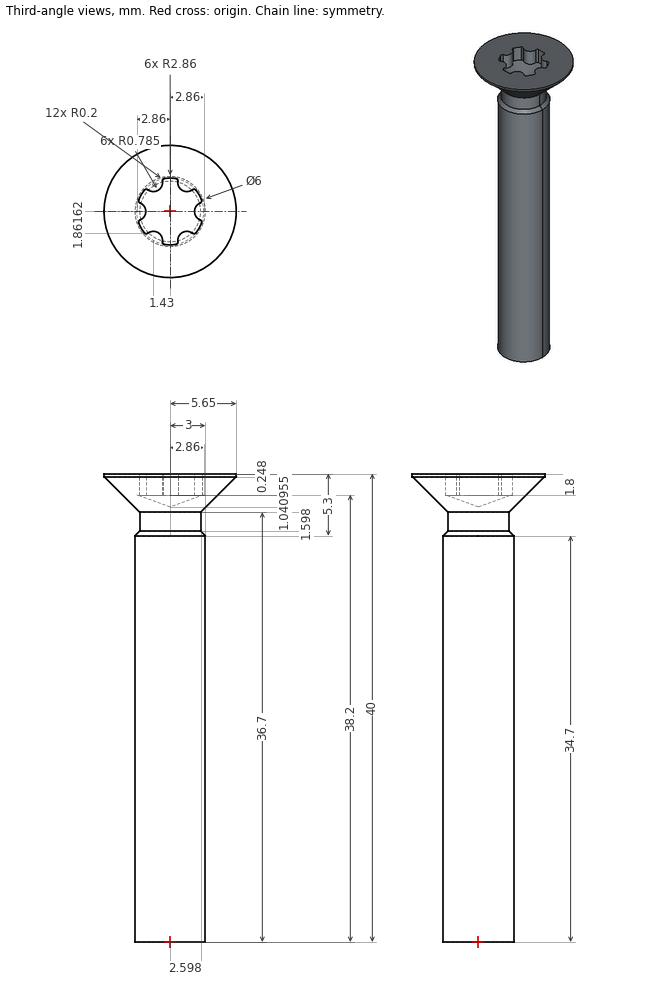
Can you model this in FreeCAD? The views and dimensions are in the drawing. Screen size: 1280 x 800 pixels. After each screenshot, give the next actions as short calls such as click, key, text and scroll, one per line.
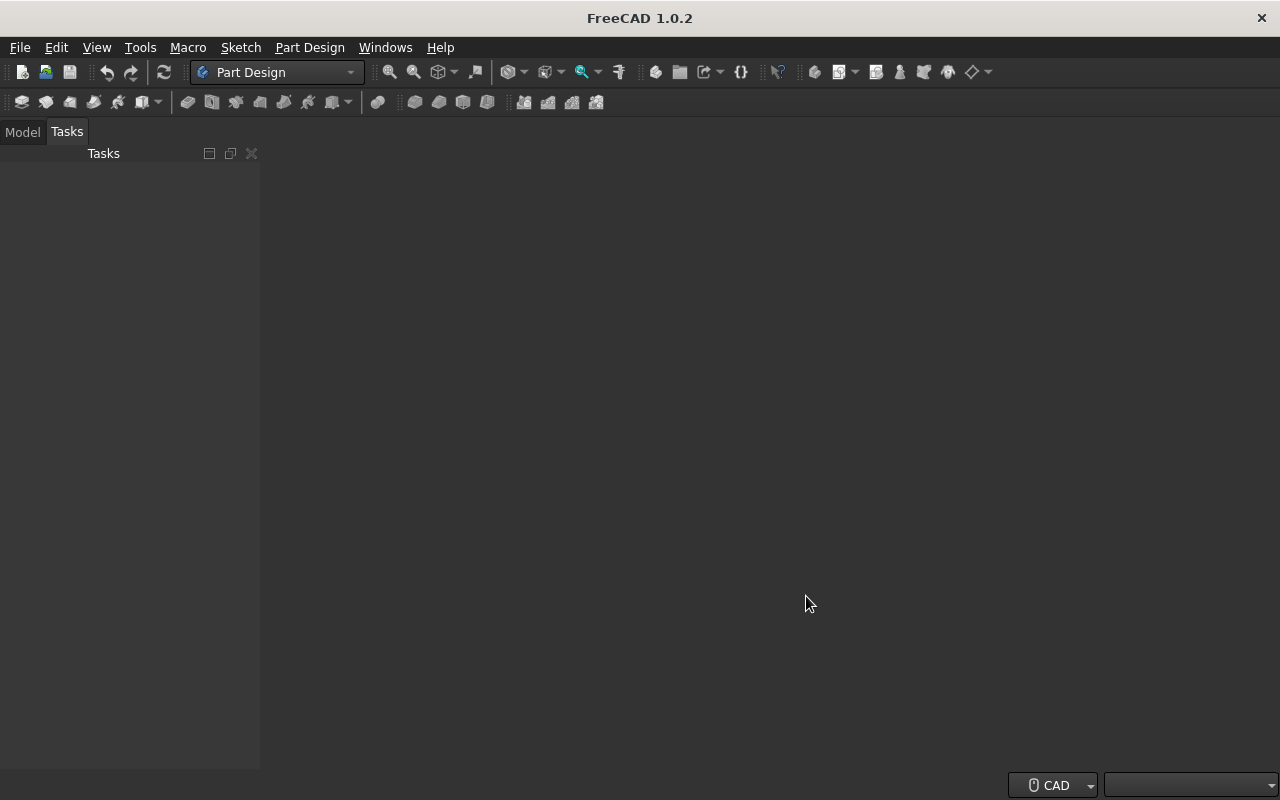
click(22, 72)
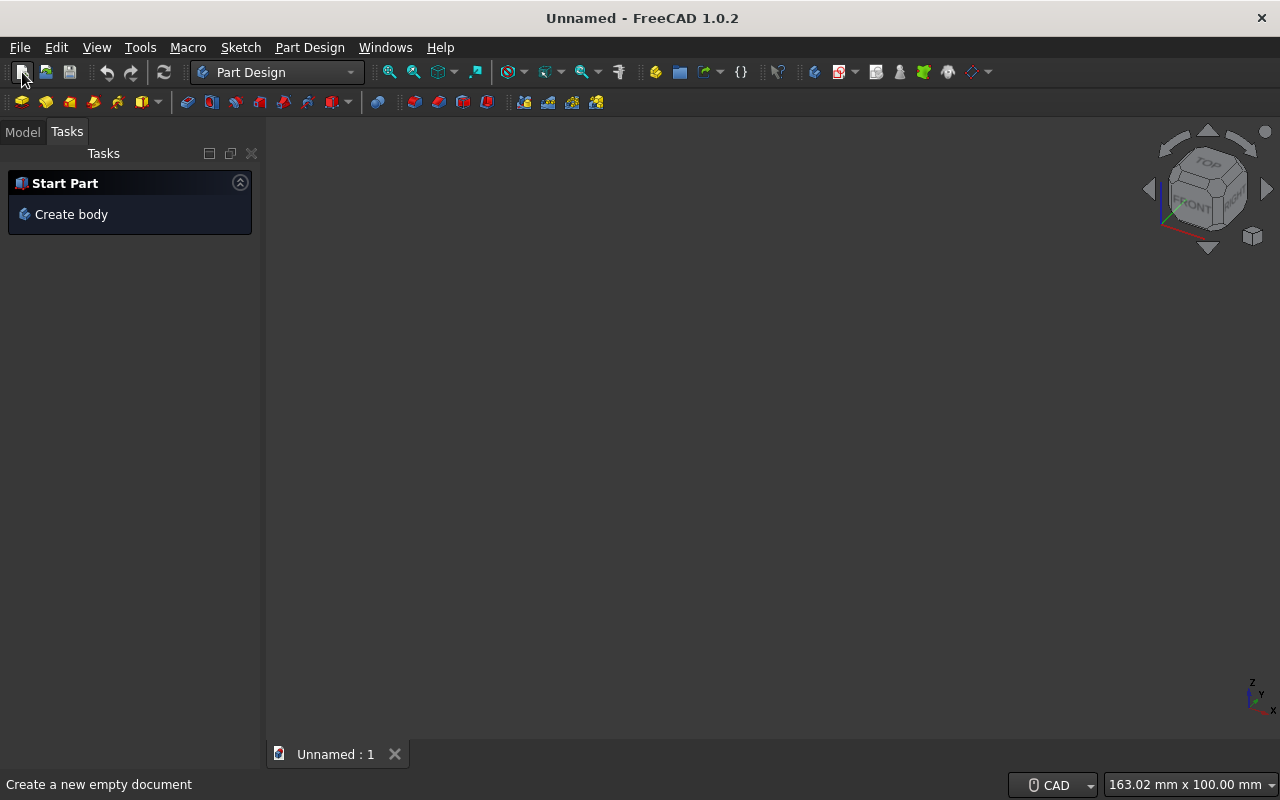
click(840, 72)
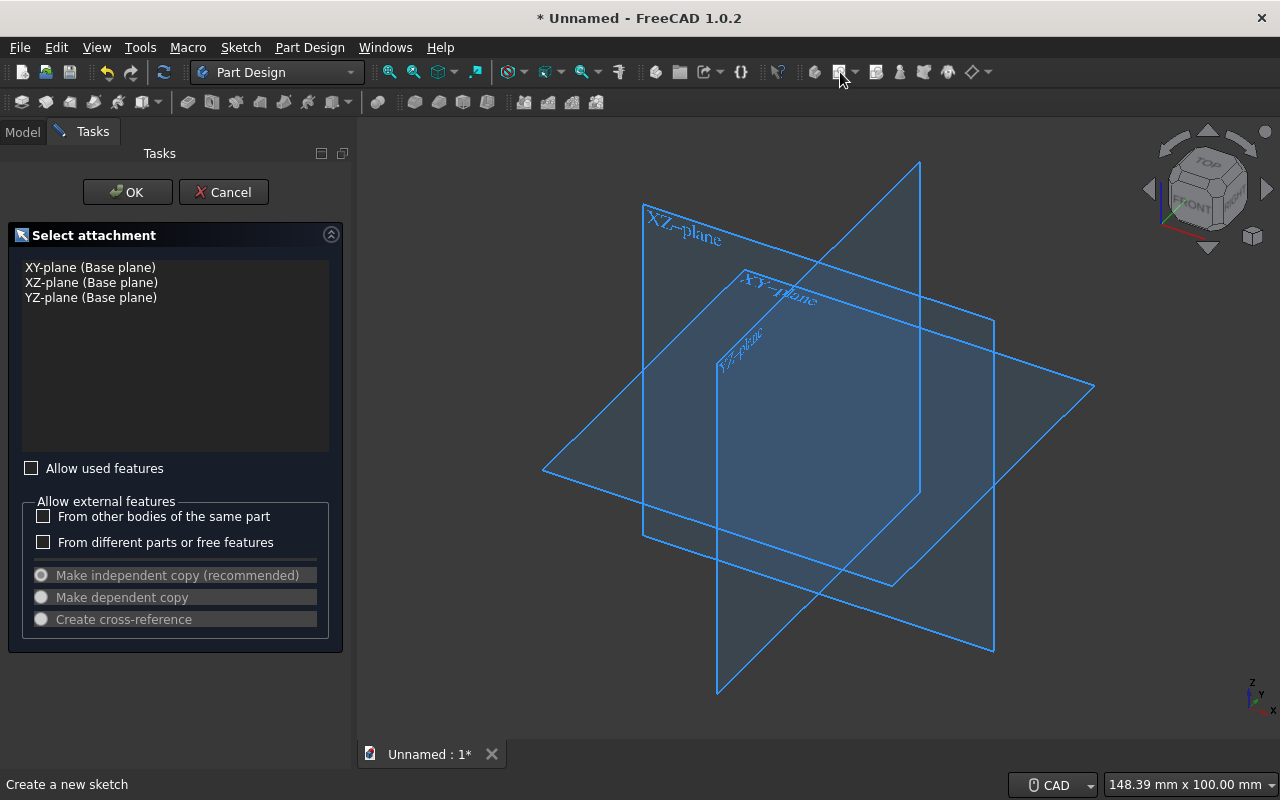
click(82, 268)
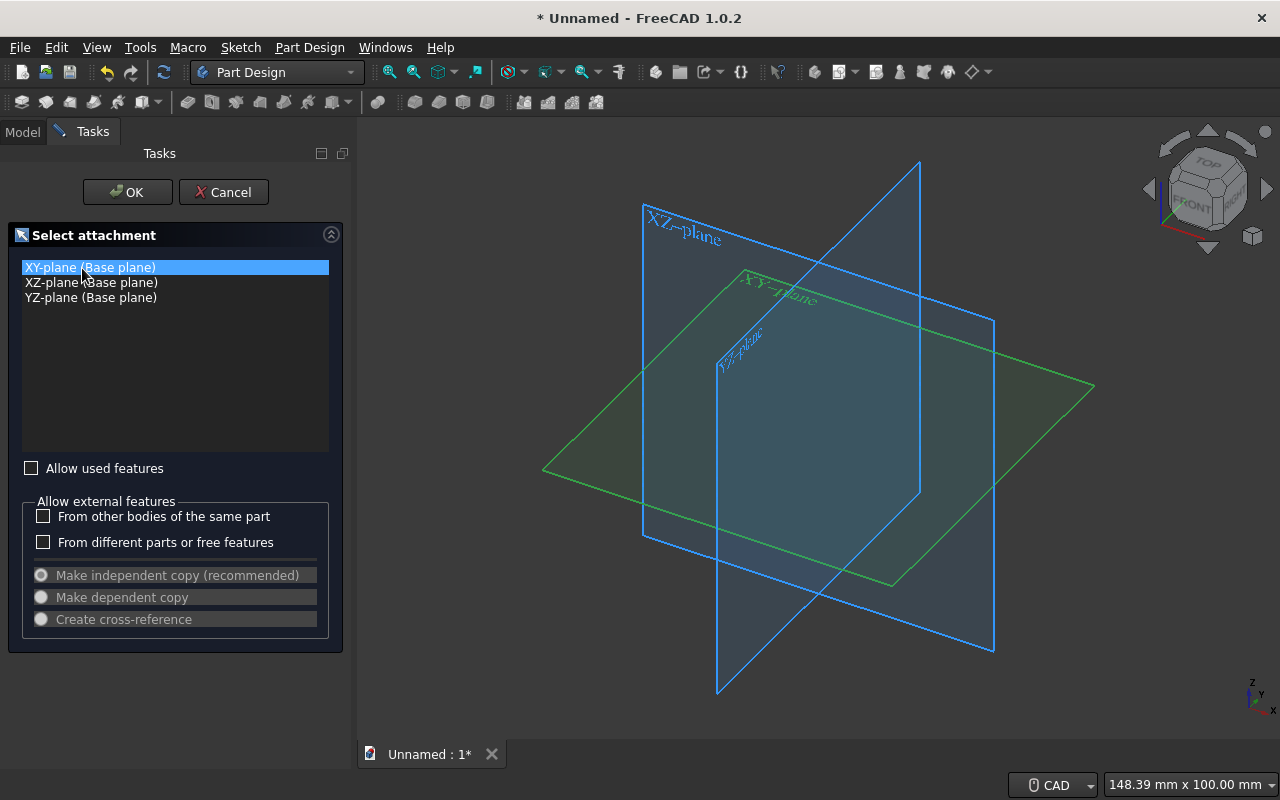
click(128, 192)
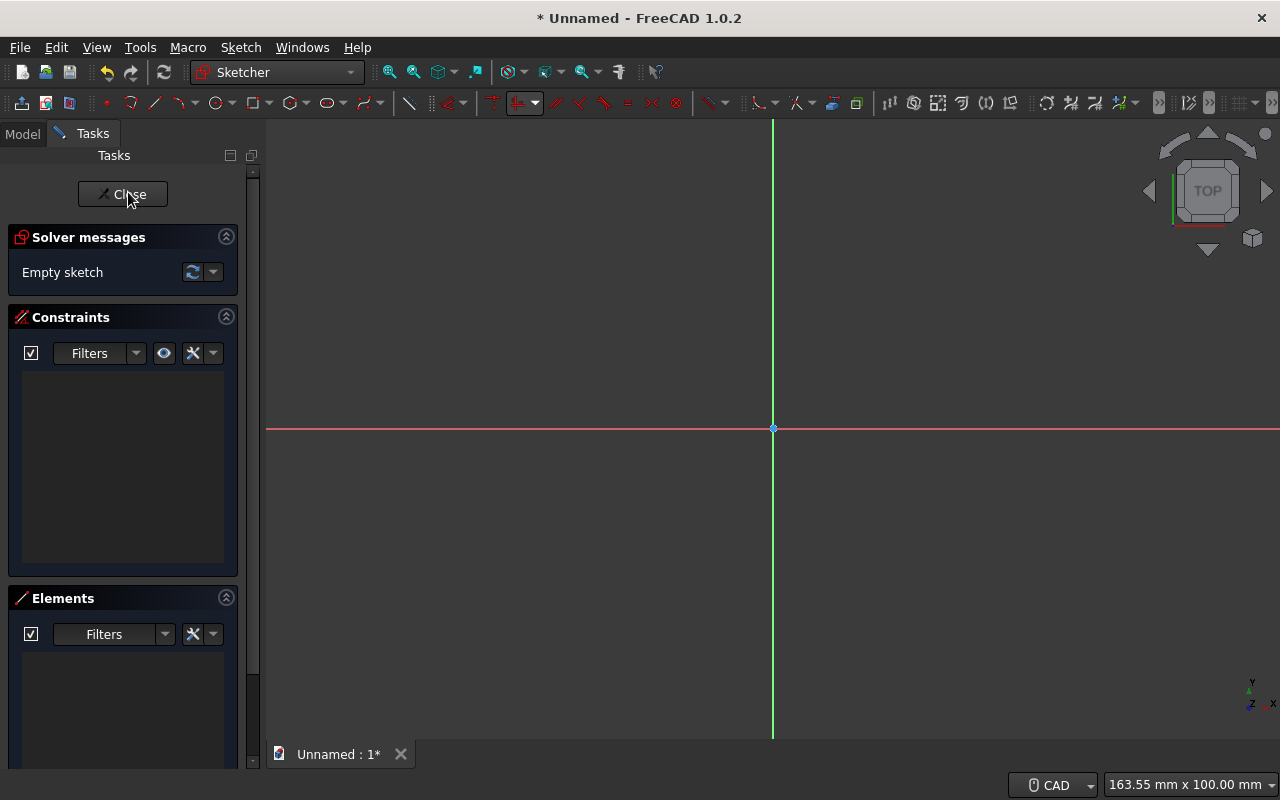
scroll(780, 429, up, 12)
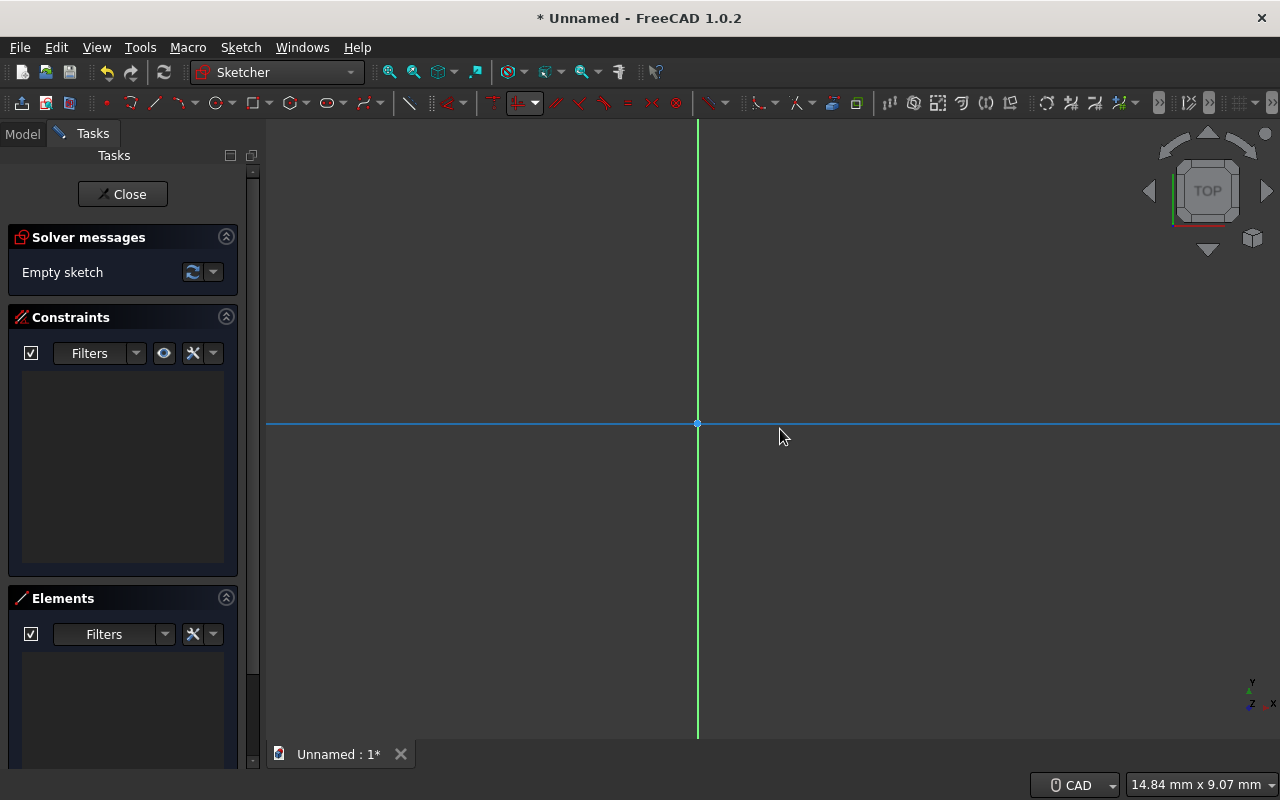
click(216, 104)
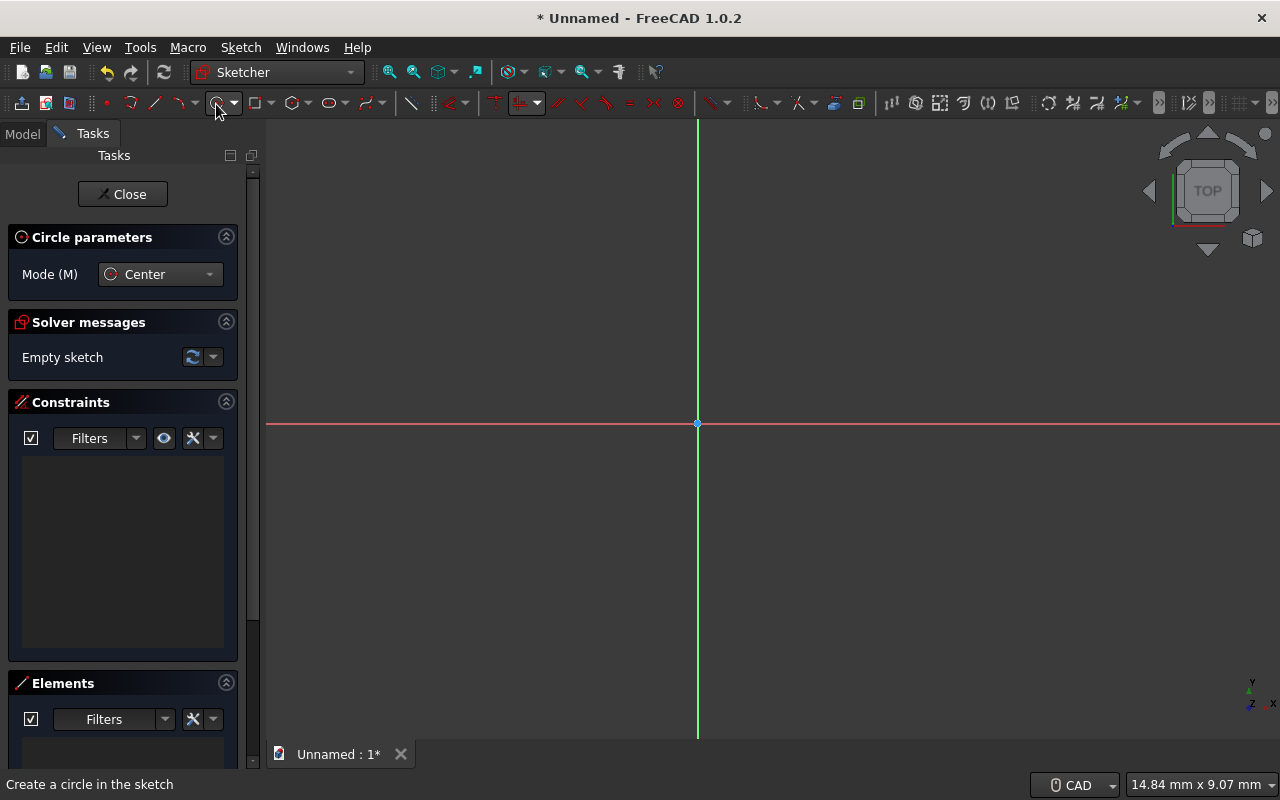
click(698, 424)
move(843, 279)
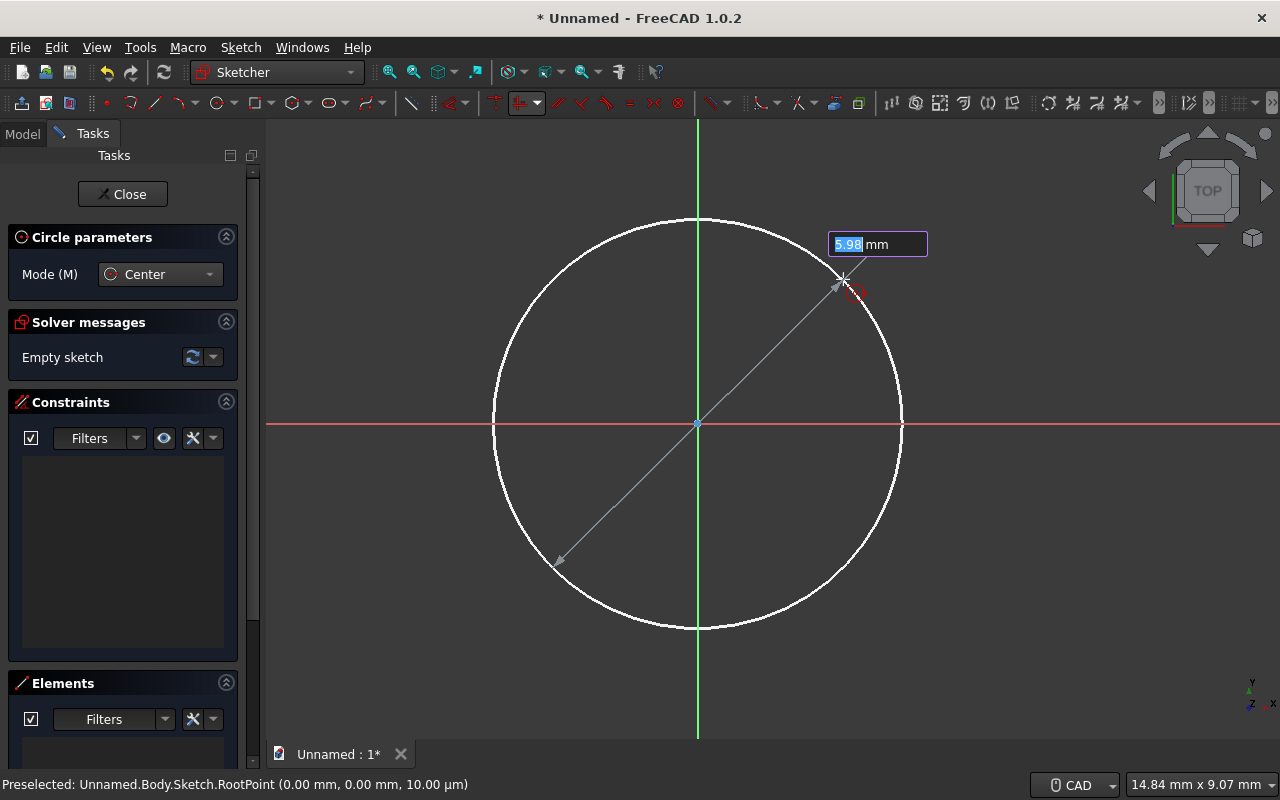
text(6)
key(Return)
key(Escape)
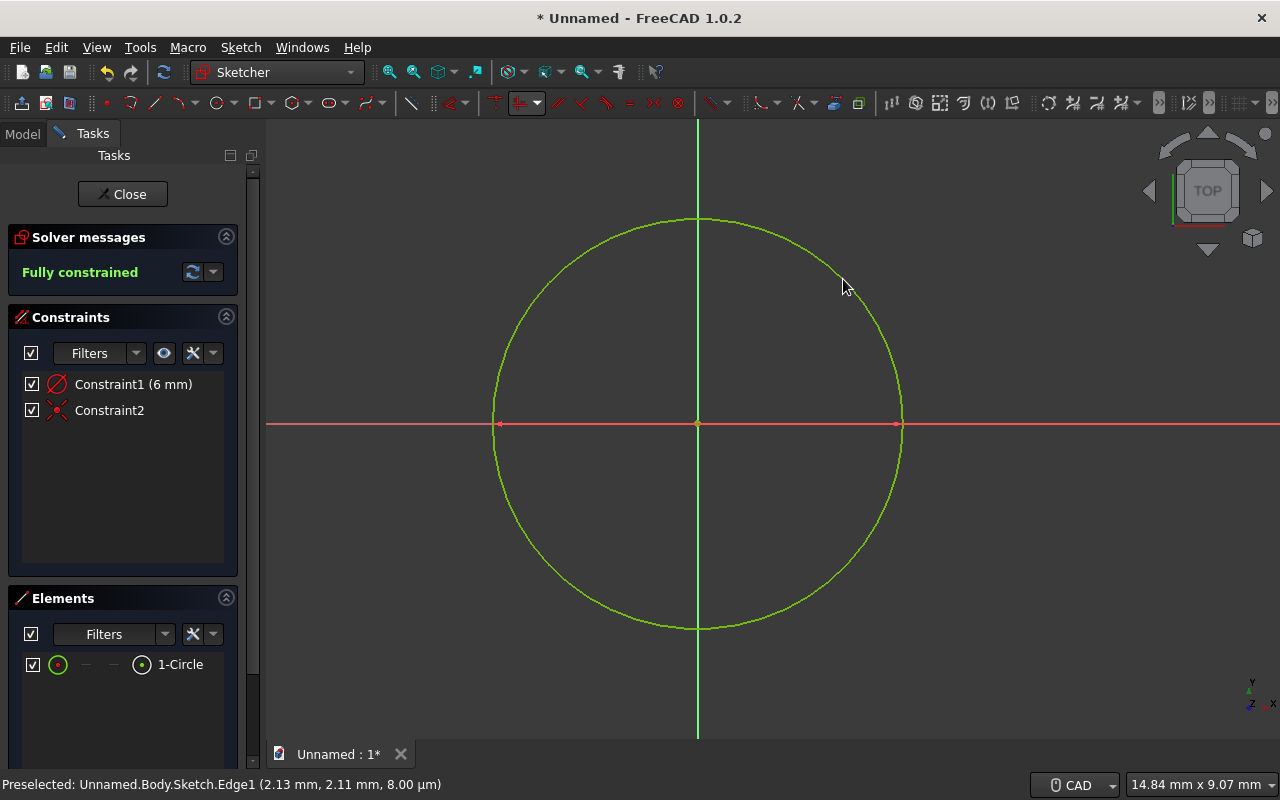
click(123, 194)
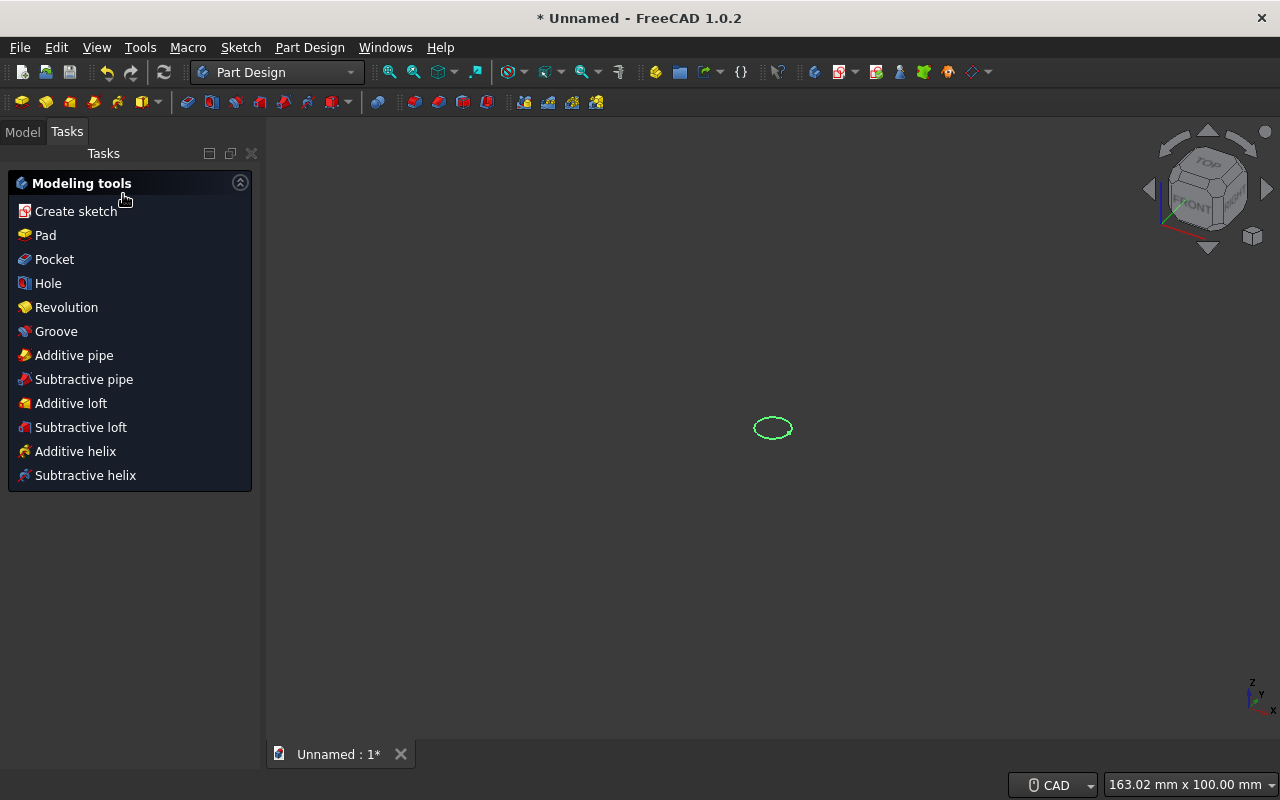
click(22, 102)